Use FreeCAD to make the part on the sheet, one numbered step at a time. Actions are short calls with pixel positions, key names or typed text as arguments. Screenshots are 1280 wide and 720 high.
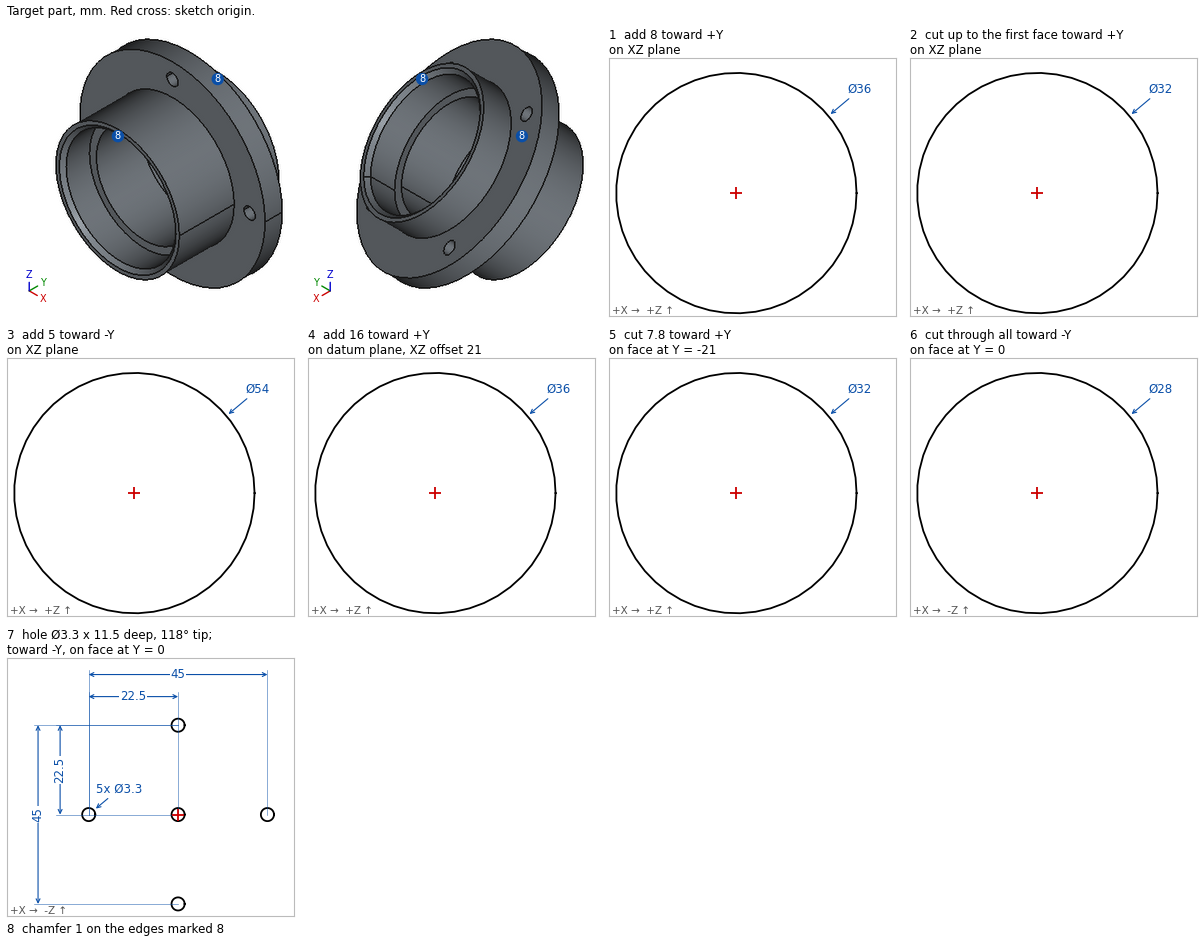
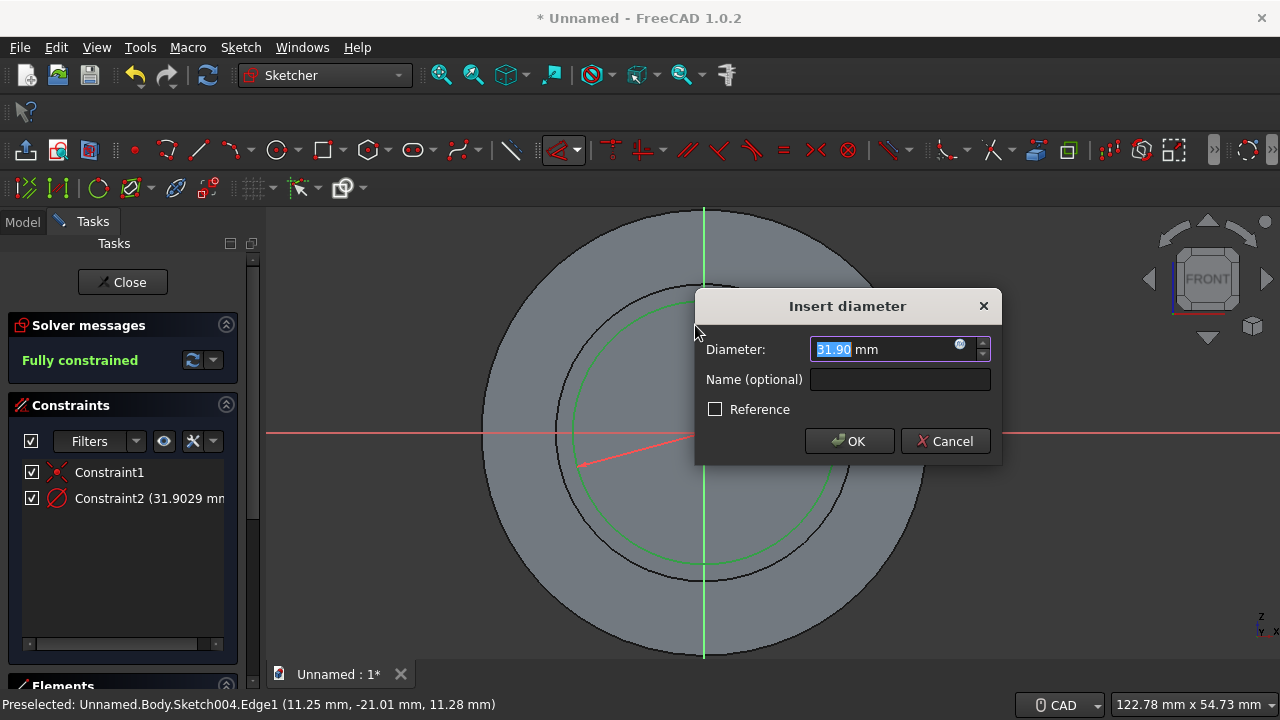
text(32)
key(Return)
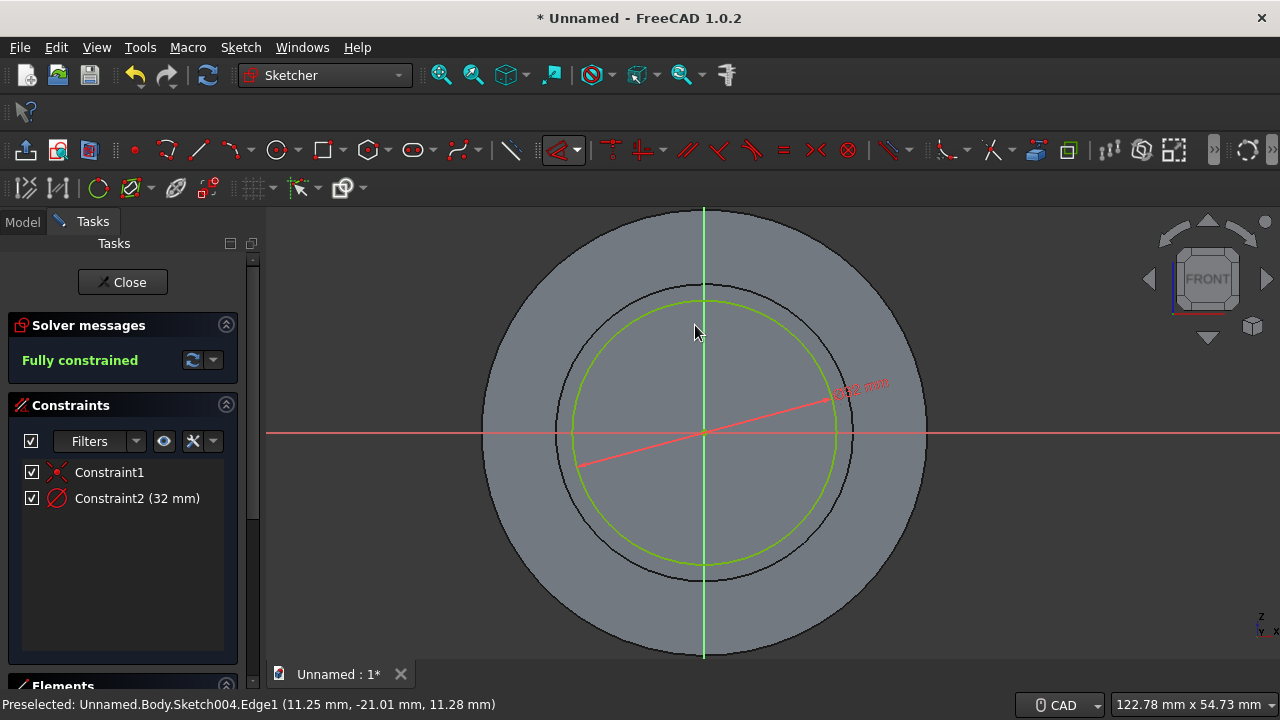
click(123, 282)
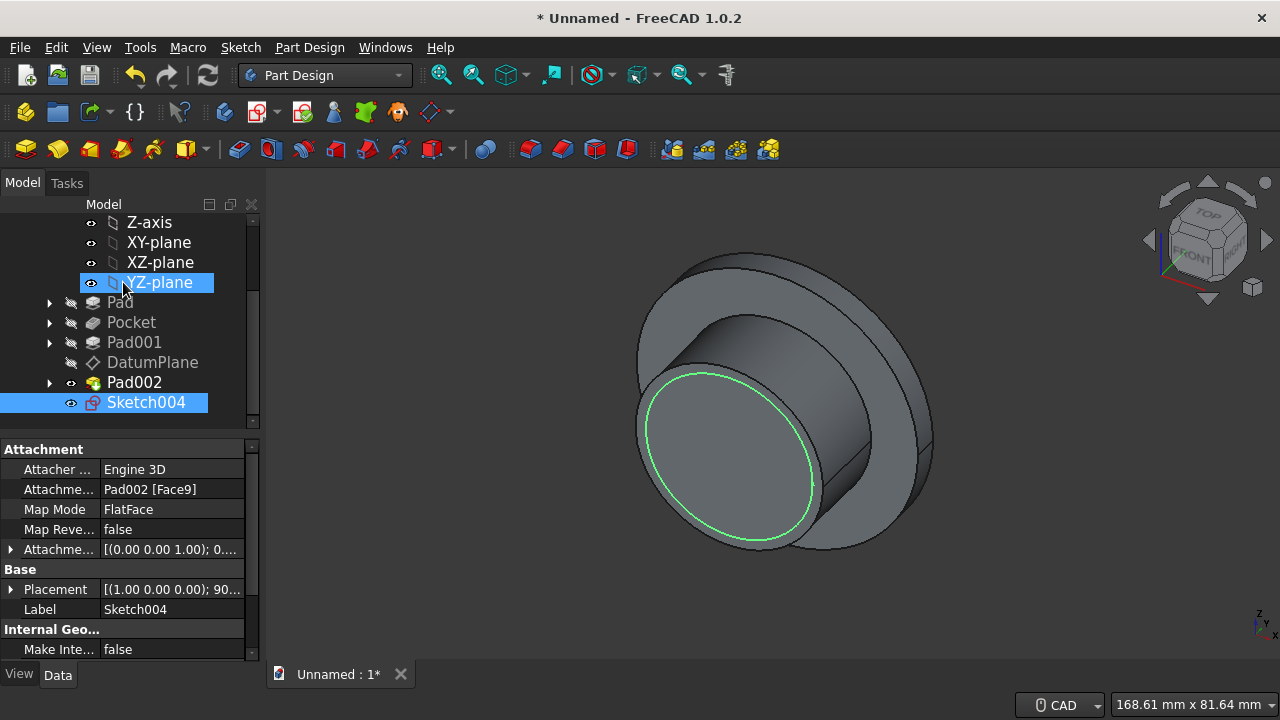
click(240, 150)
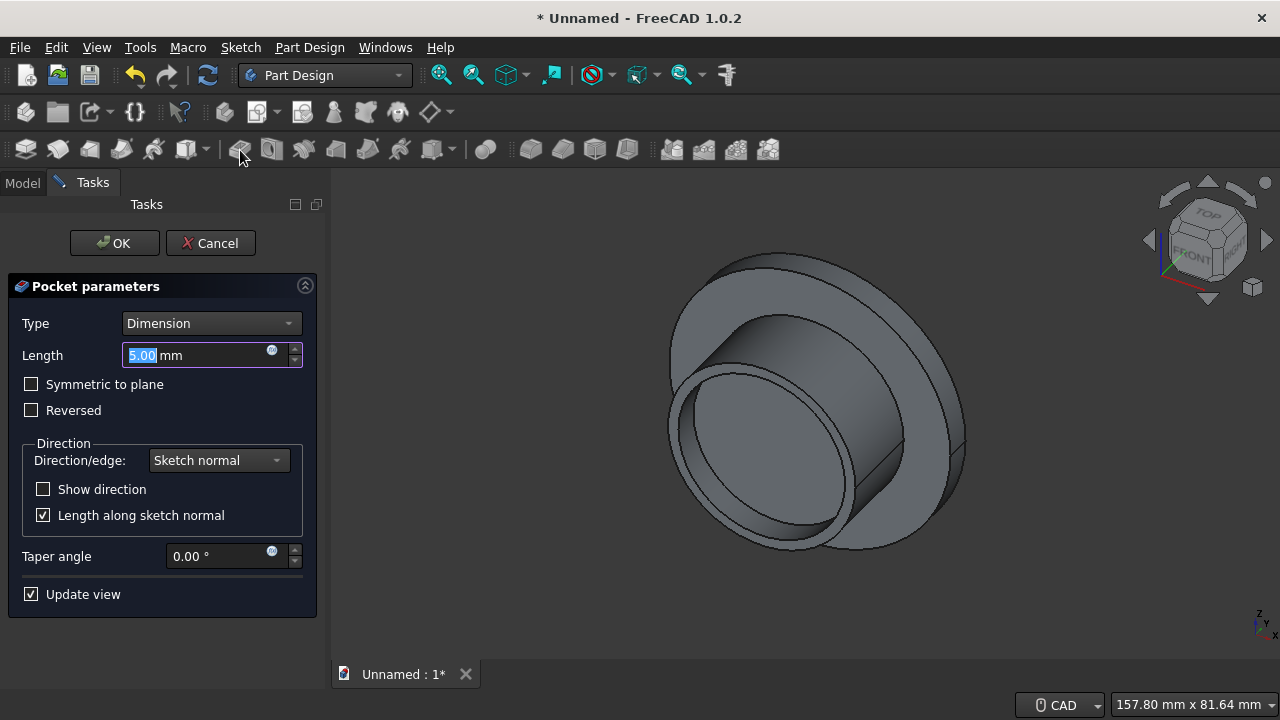
text(7.8)
key(Tab)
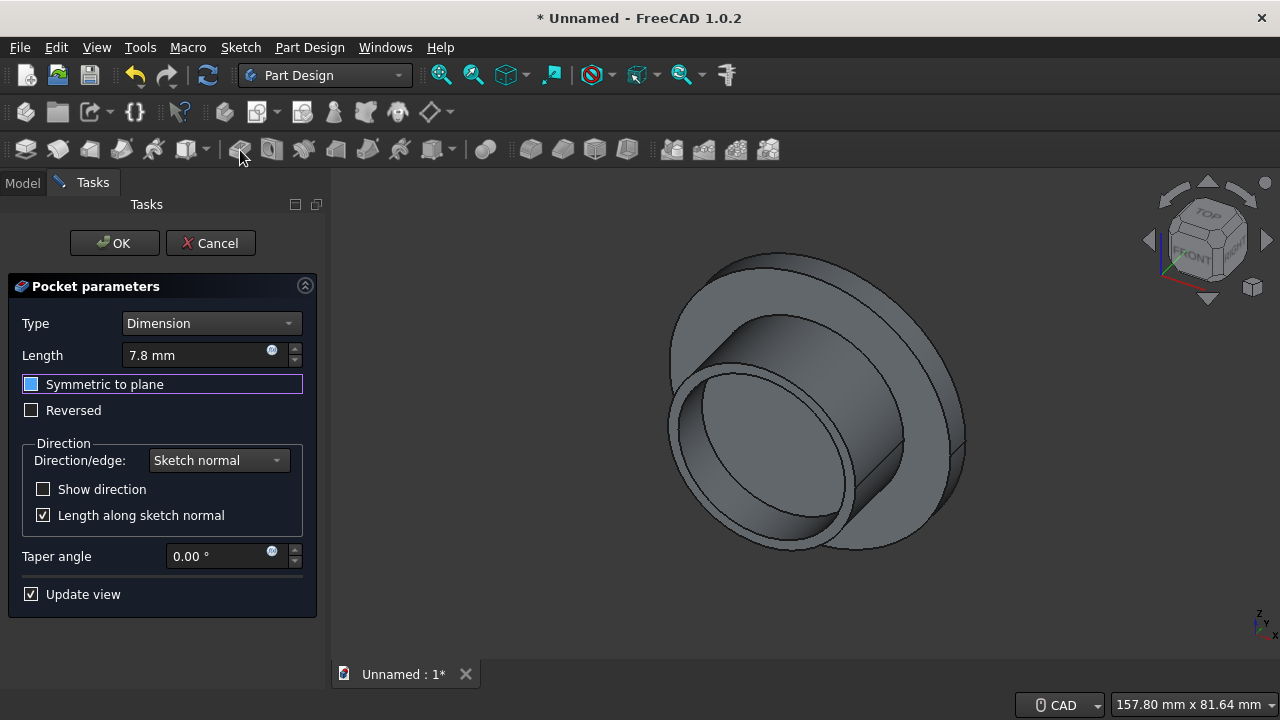
click(115, 243)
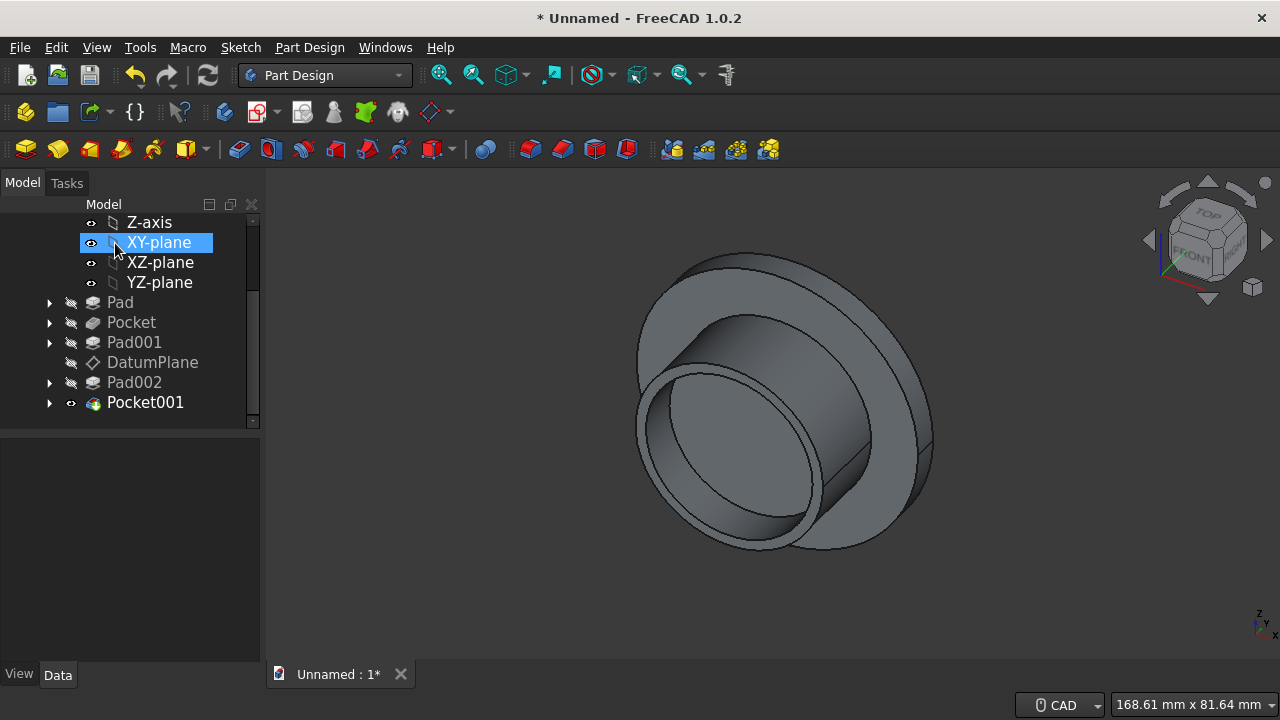
key(4)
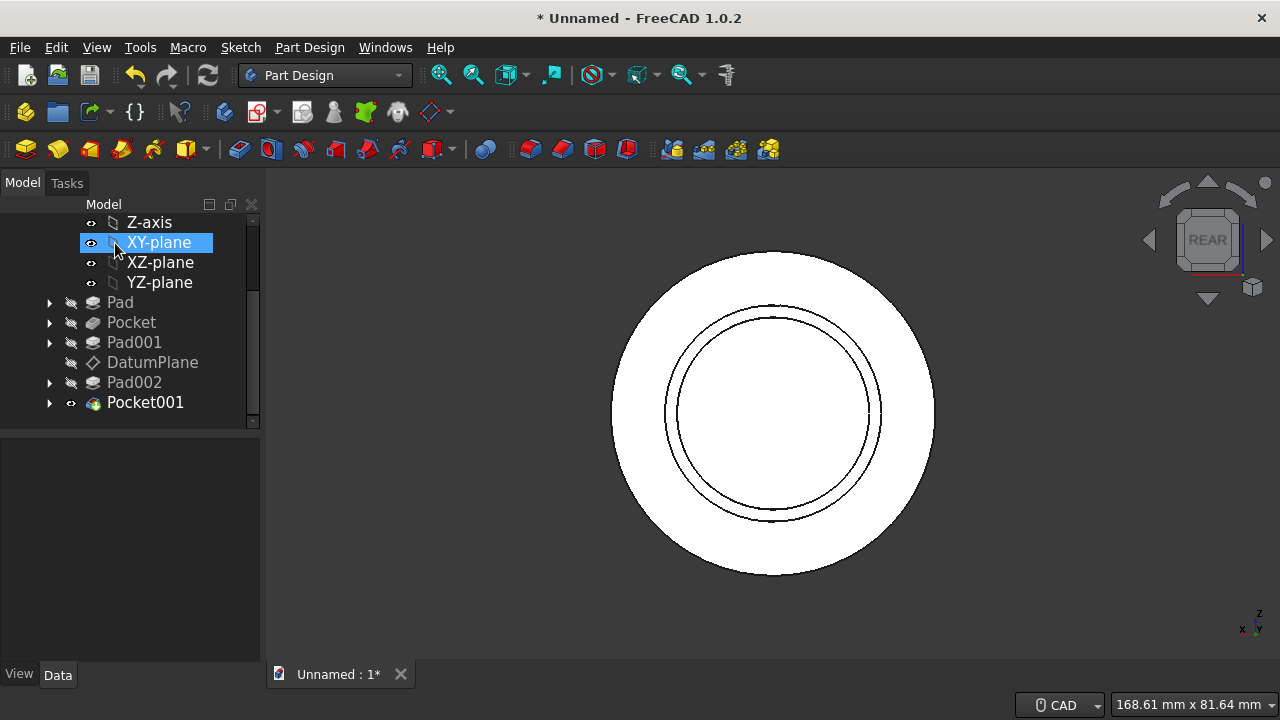
click(773, 552)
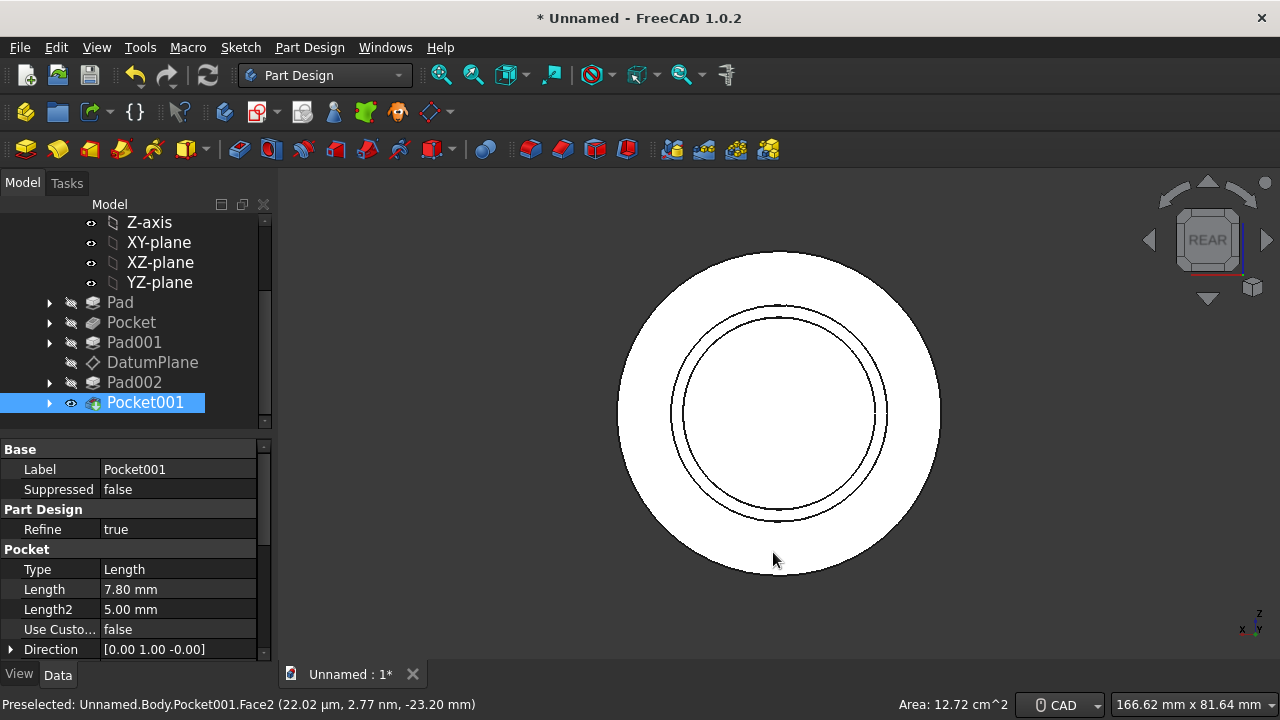
click(258, 112)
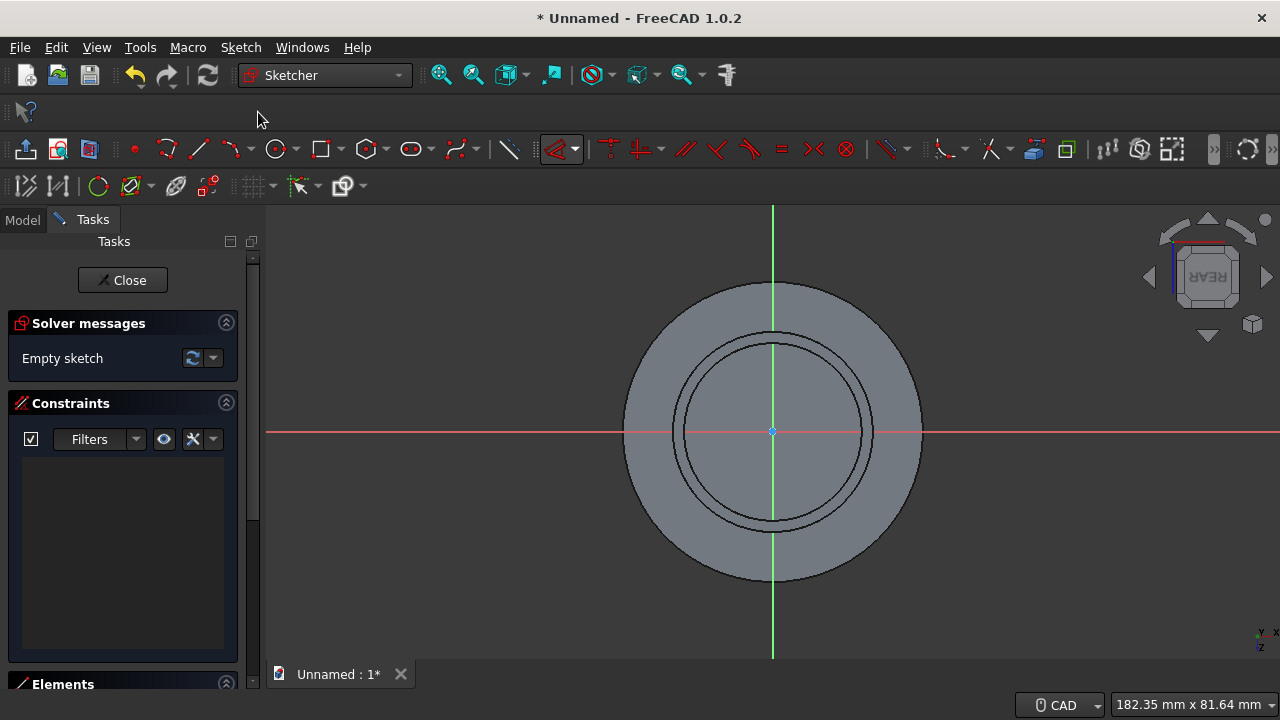
click(90, 150)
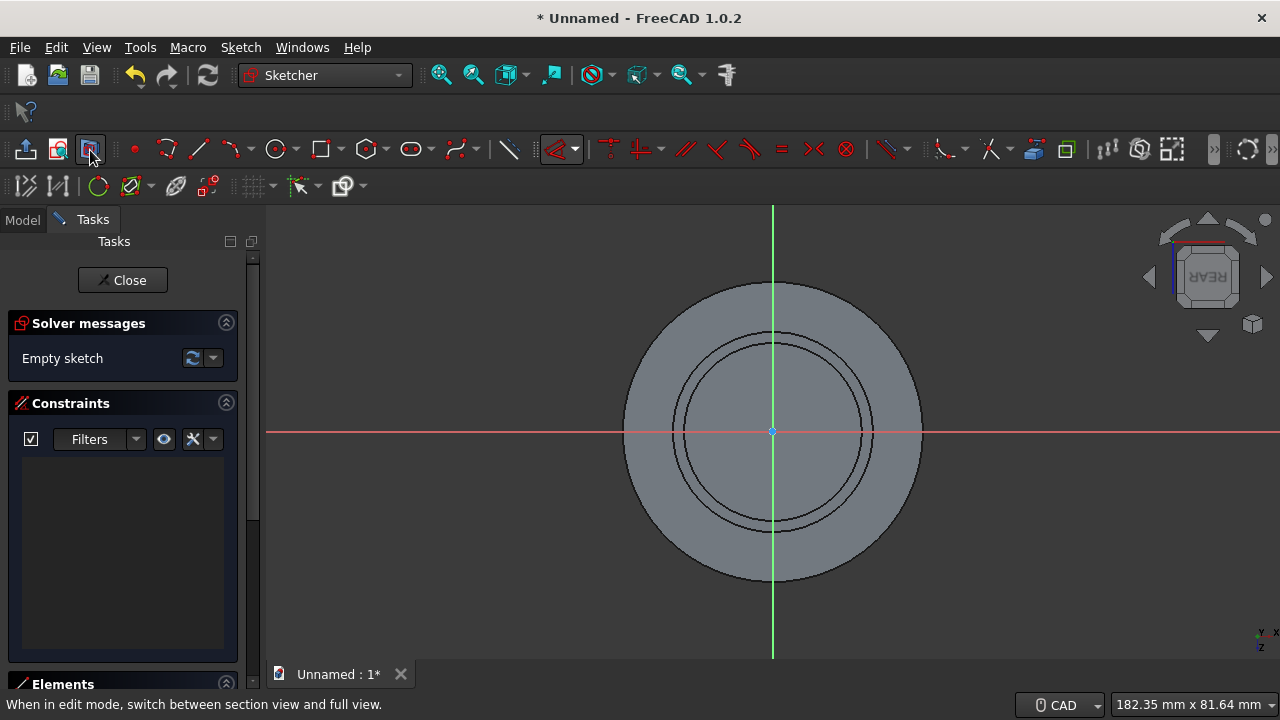
scroll(856, 432, up, 3)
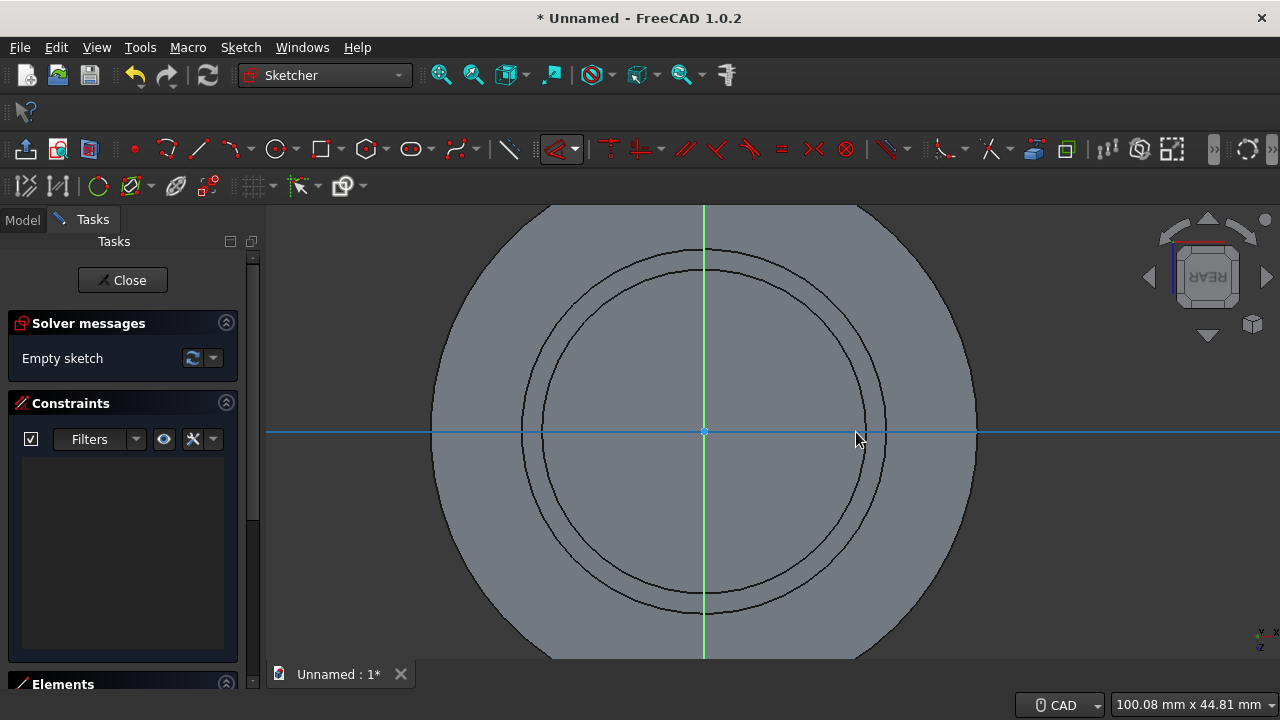
click(276, 150)